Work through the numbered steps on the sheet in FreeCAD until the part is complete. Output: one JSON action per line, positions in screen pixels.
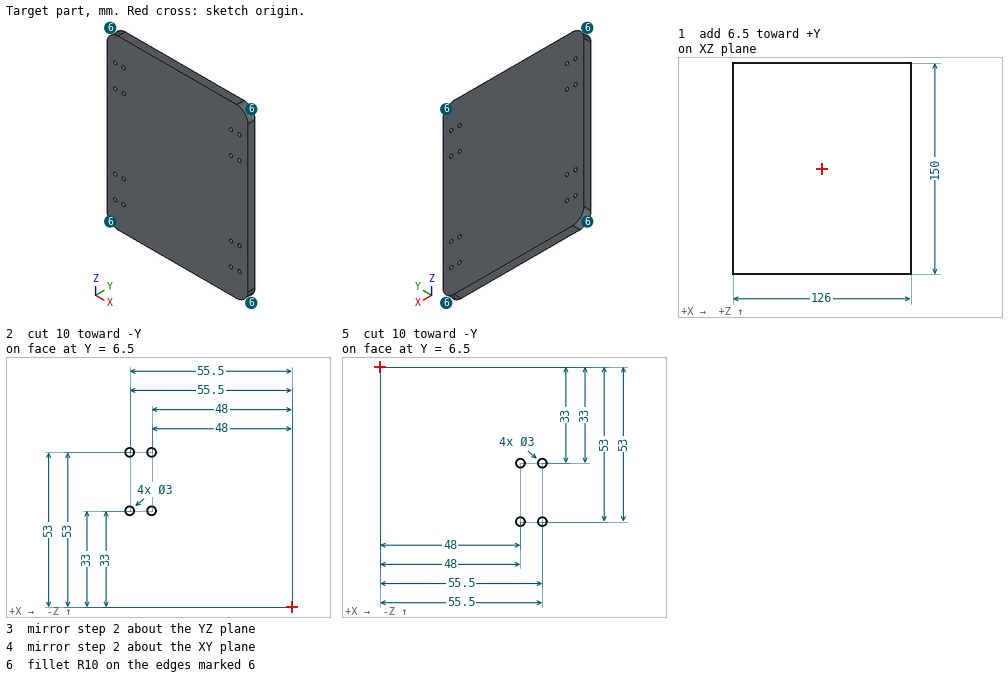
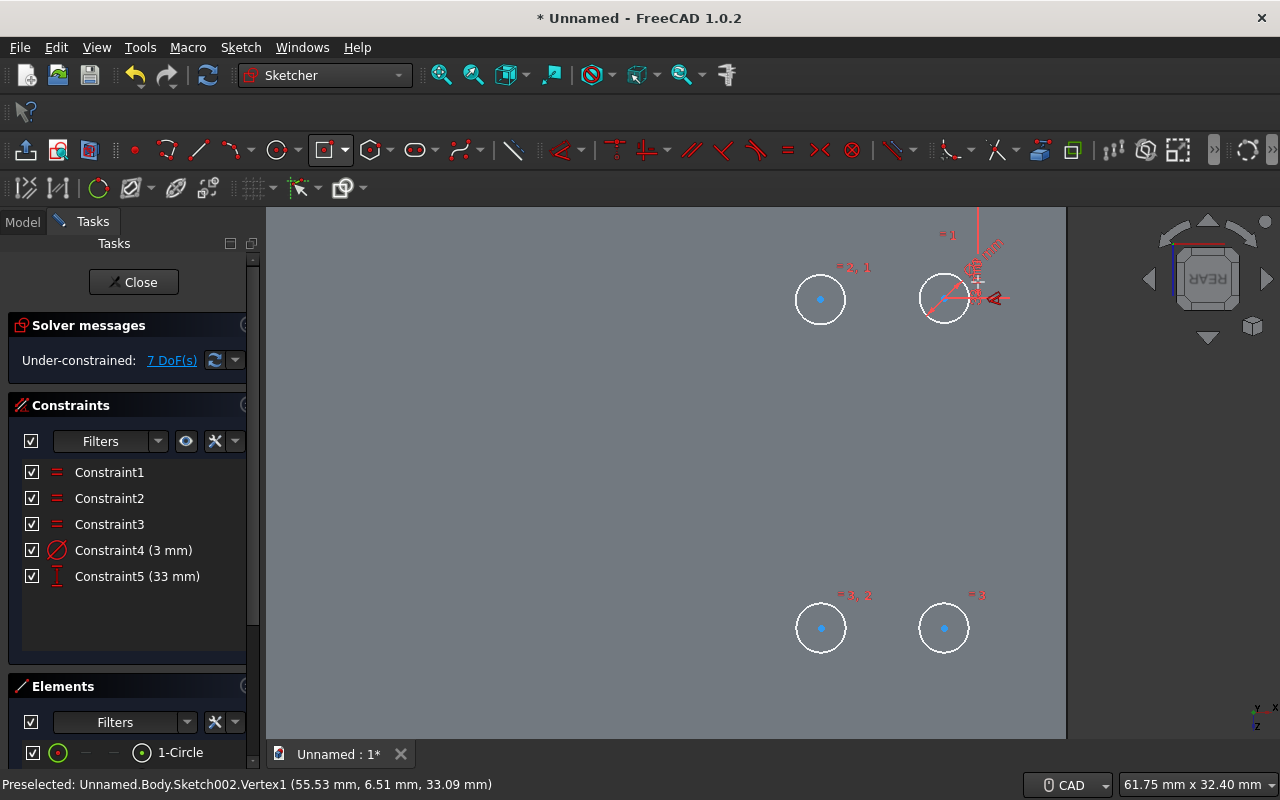
{"action": "left_click", "coordinate": [820, 300]}
{"action": "left_click", "coordinate": [557, 334]}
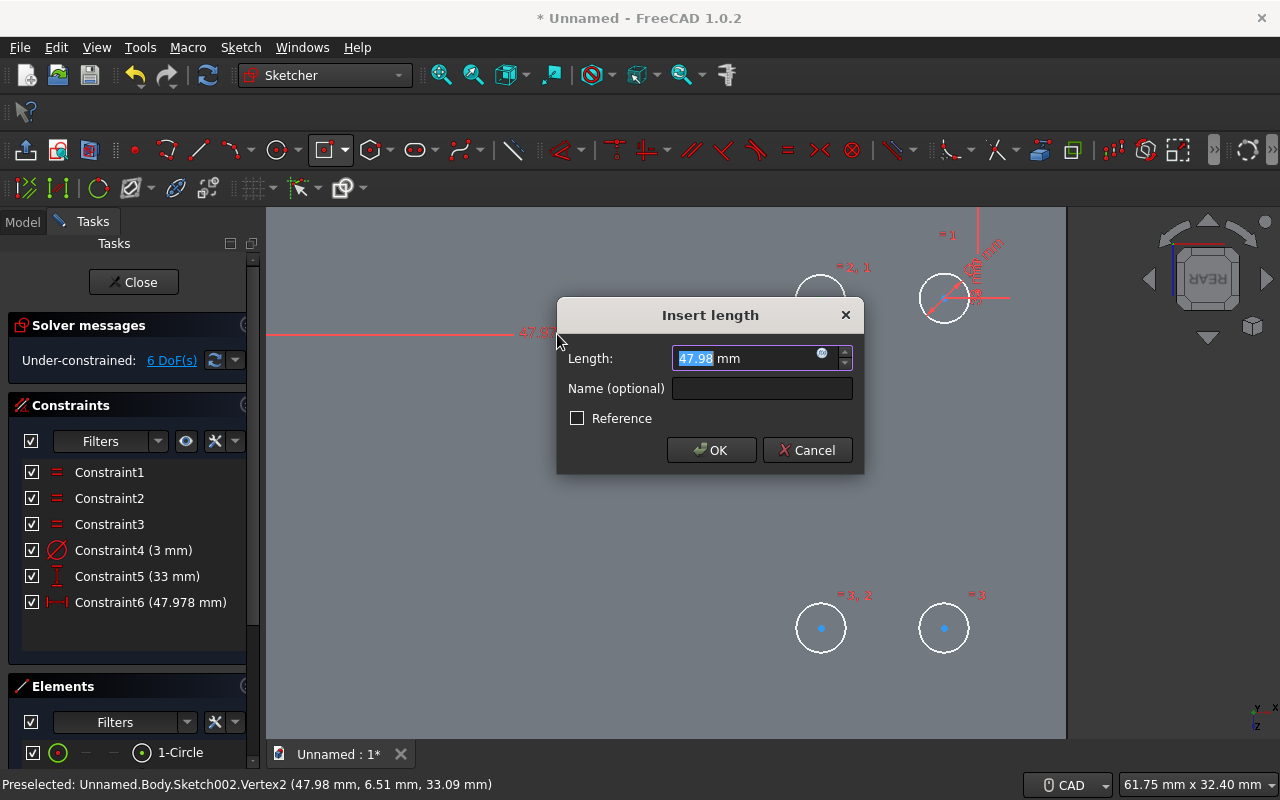
{"action": "type", "text": "48"}
{"action": "key", "text": "Return"}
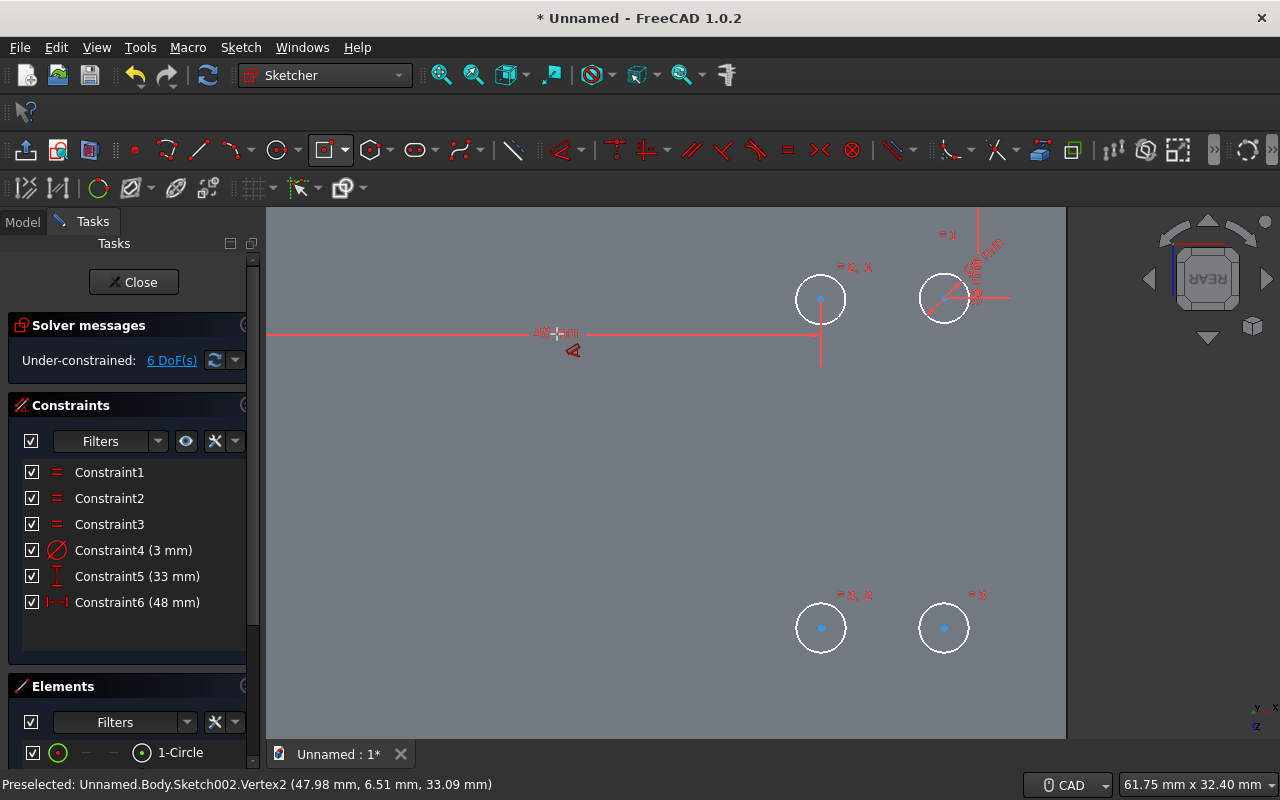
{"action": "left_click", "coordinate": [821, 300]}
{"action": "left_click", "coordinate": [855, 267]}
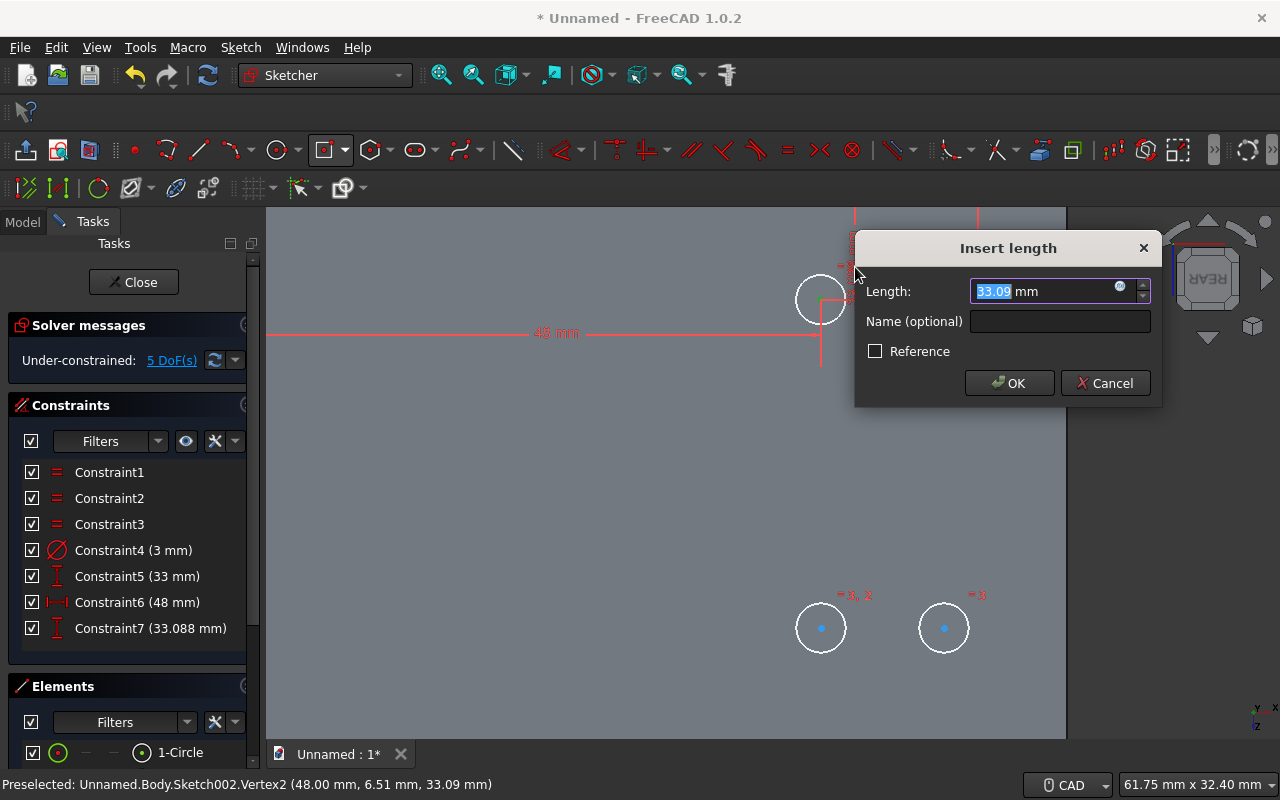
{"action": "type", "text": "33"}
{"action": "key", "text": "Return"}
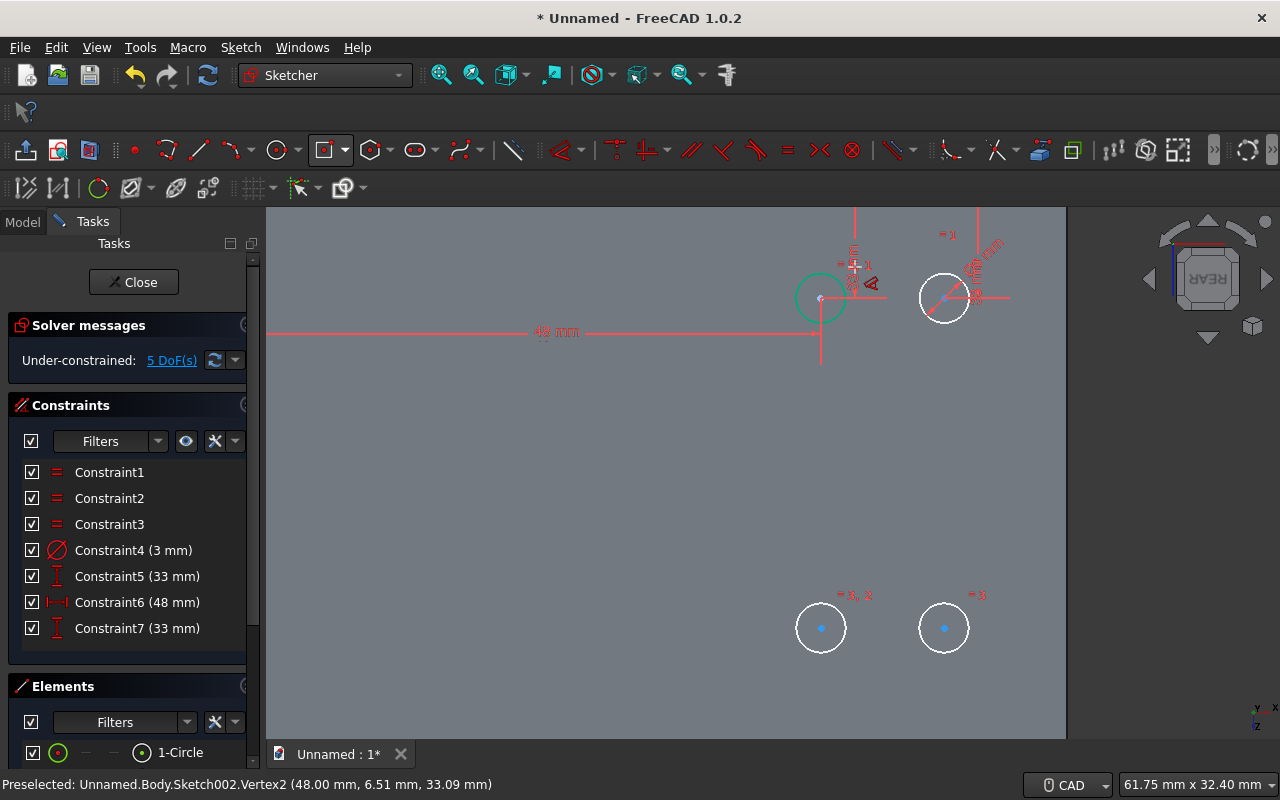
{"action": "left_click", "coordinate": [821, 628]}
{"action": "left_click", "coordinate": [558, 662]}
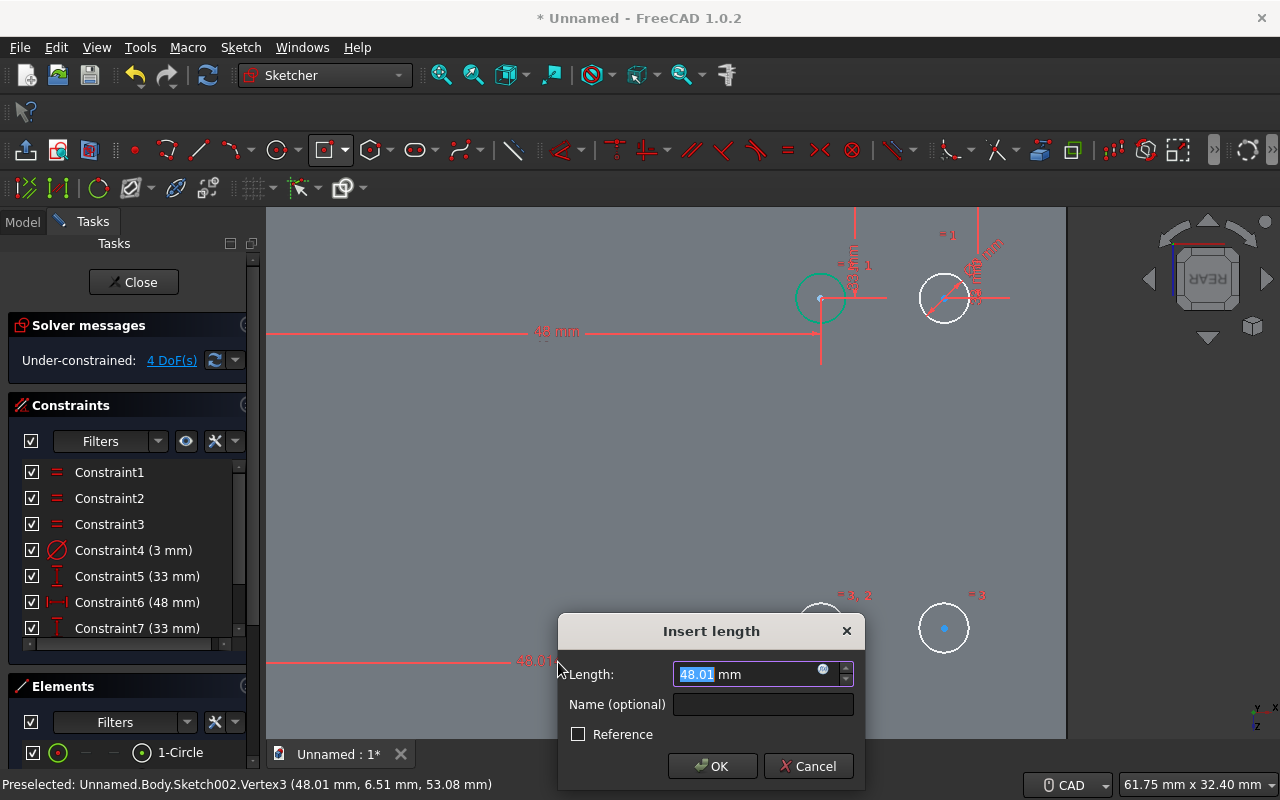
{"action": "type", "text": "48"}
{"action": "key", "text": "Return"}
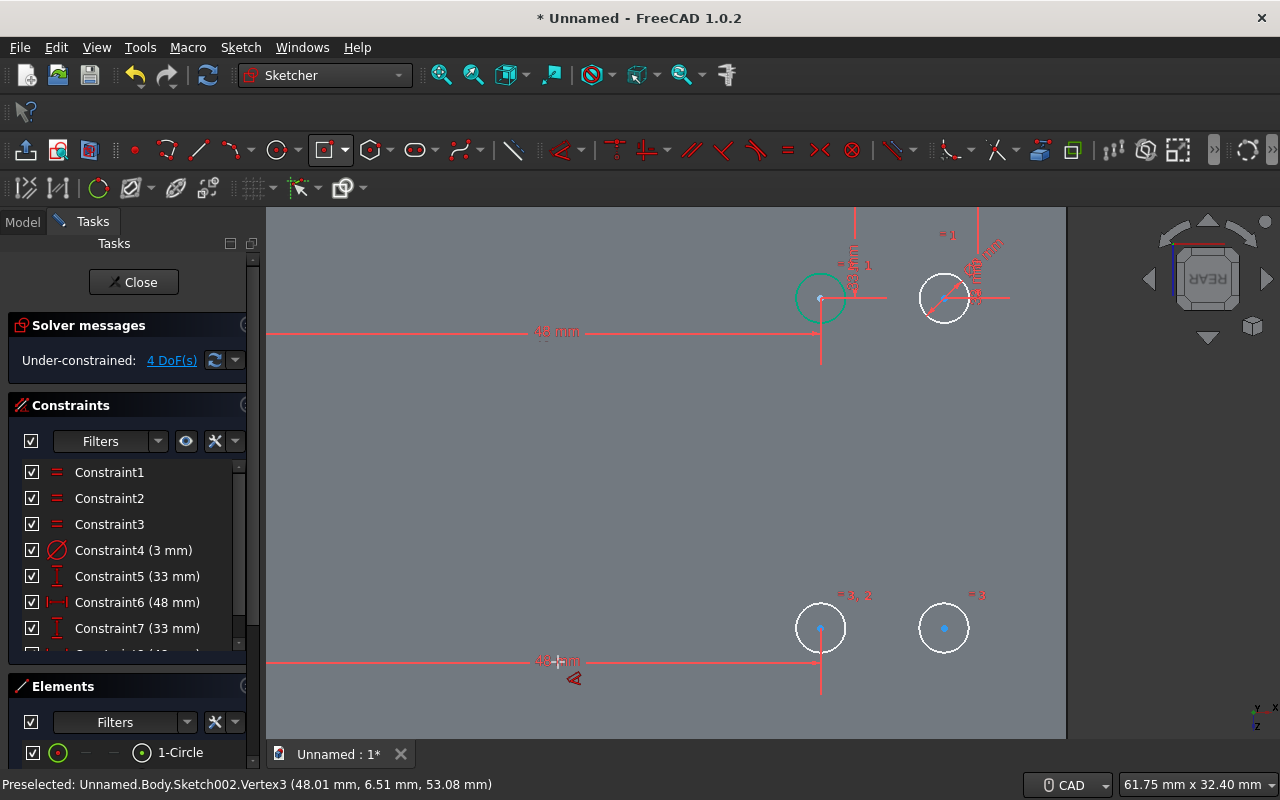
{"action": "left_click", "coordinate": [821, 628]}
{"action": "left_click", "coordinate": [855, 432]}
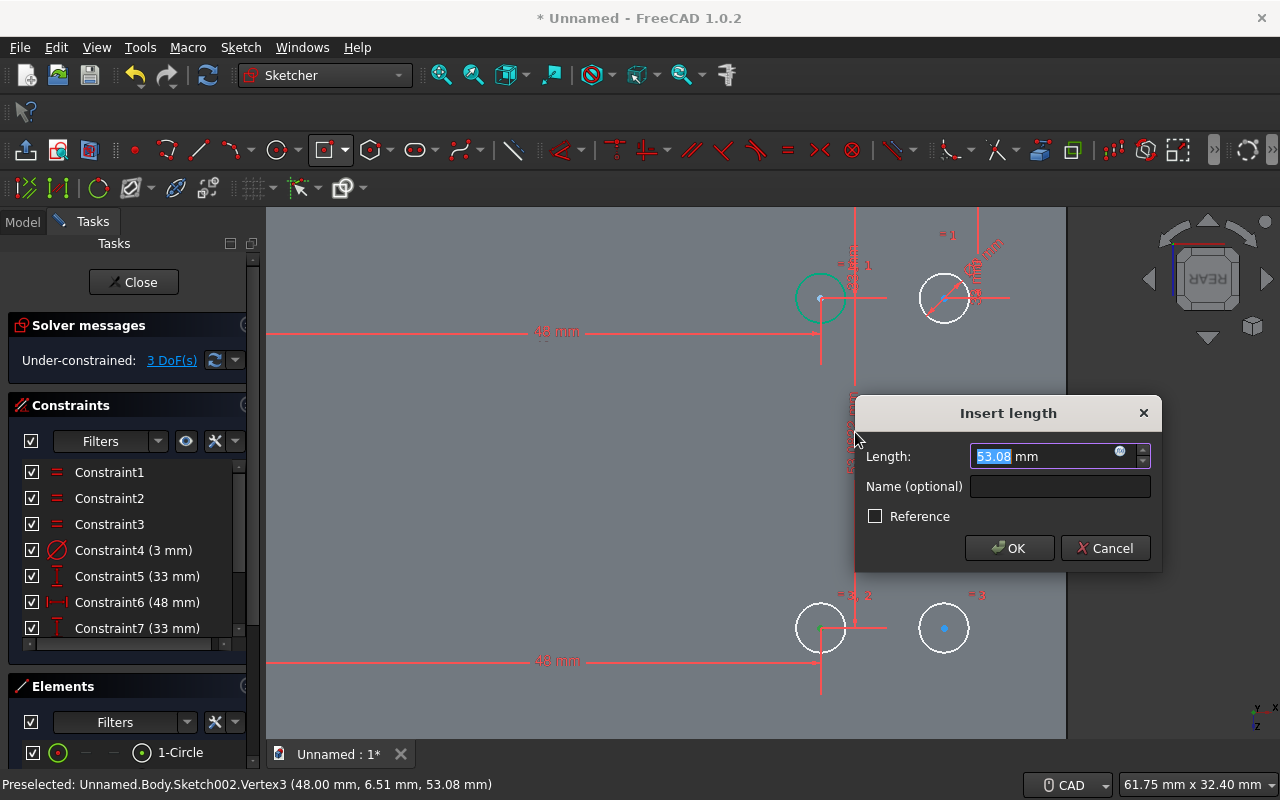
{"action": "type", "text": "53"}
{"action": "key", "text": "Return"}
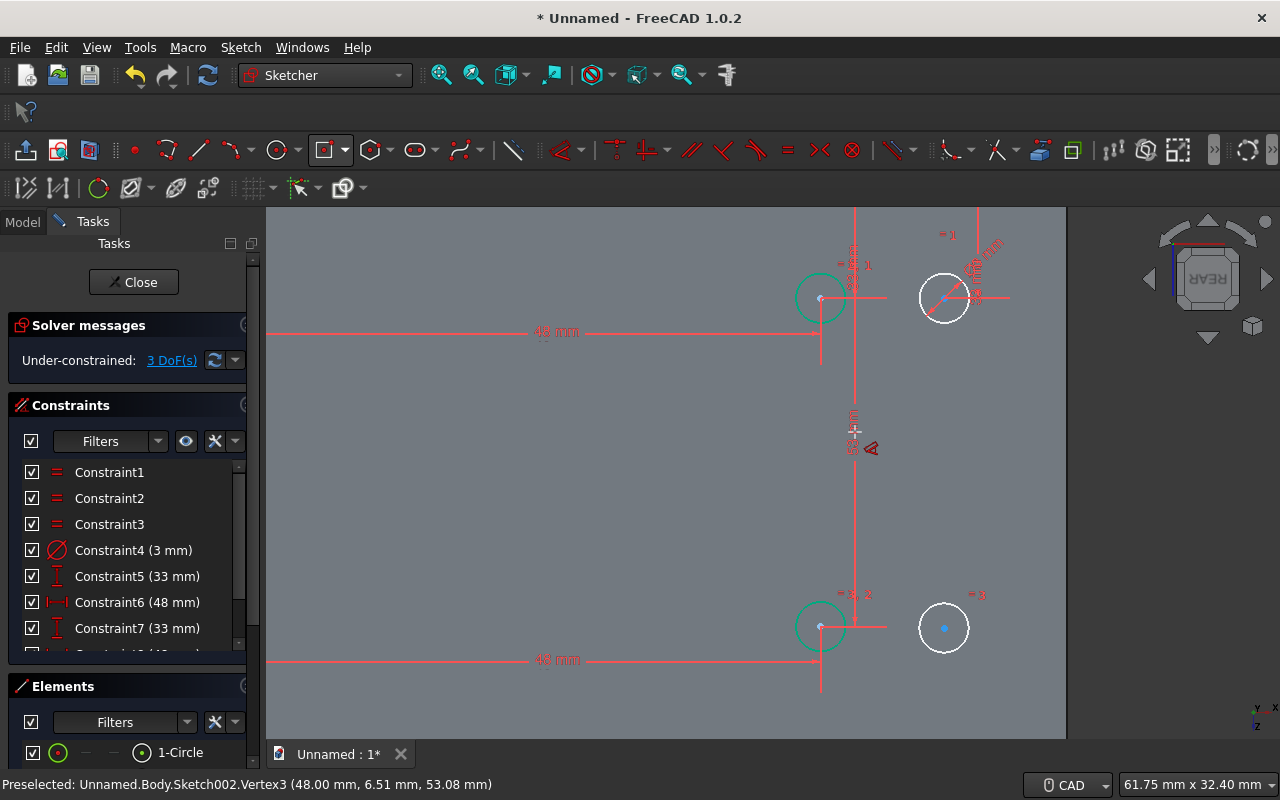
{"action": "left_click", "coordinate": [944, 628]}
{"action": "left_click", "coordinate": [978, 432]}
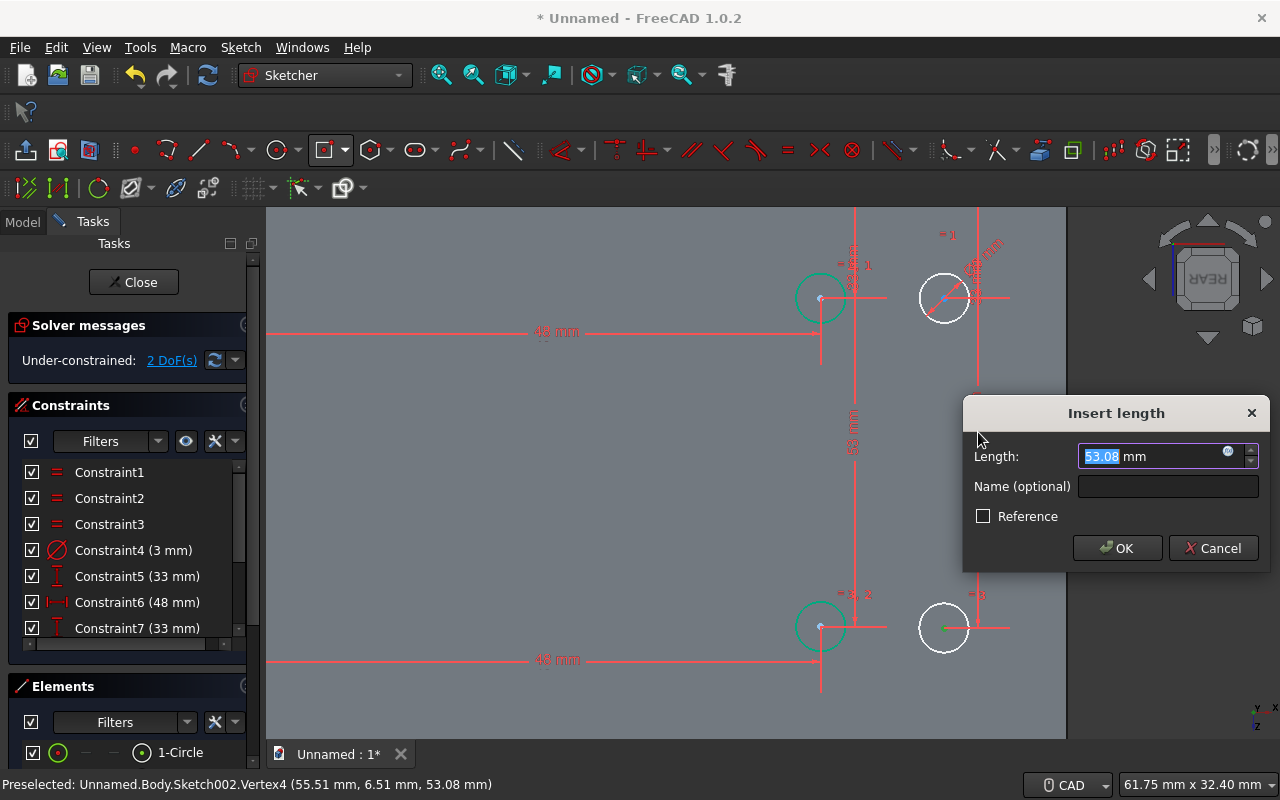
{"action": "type", "text": "53"}
{"action": "key", "text": "Return"}